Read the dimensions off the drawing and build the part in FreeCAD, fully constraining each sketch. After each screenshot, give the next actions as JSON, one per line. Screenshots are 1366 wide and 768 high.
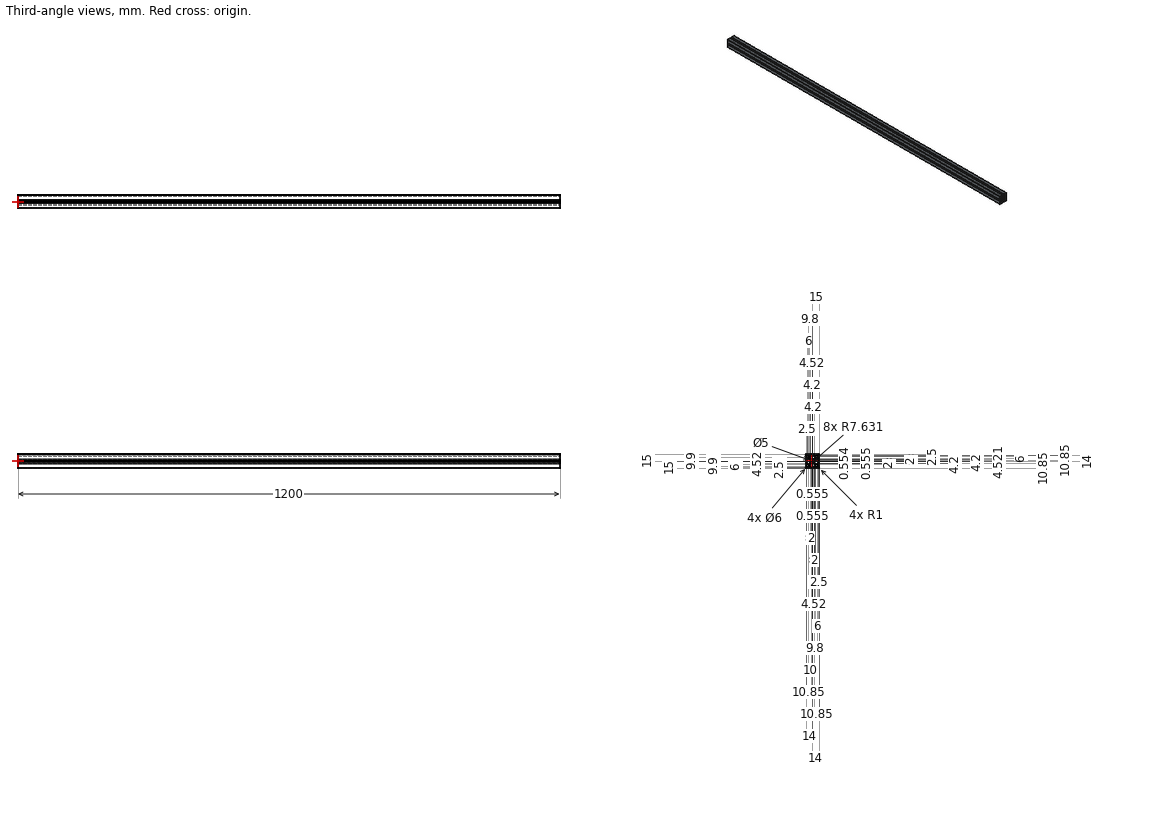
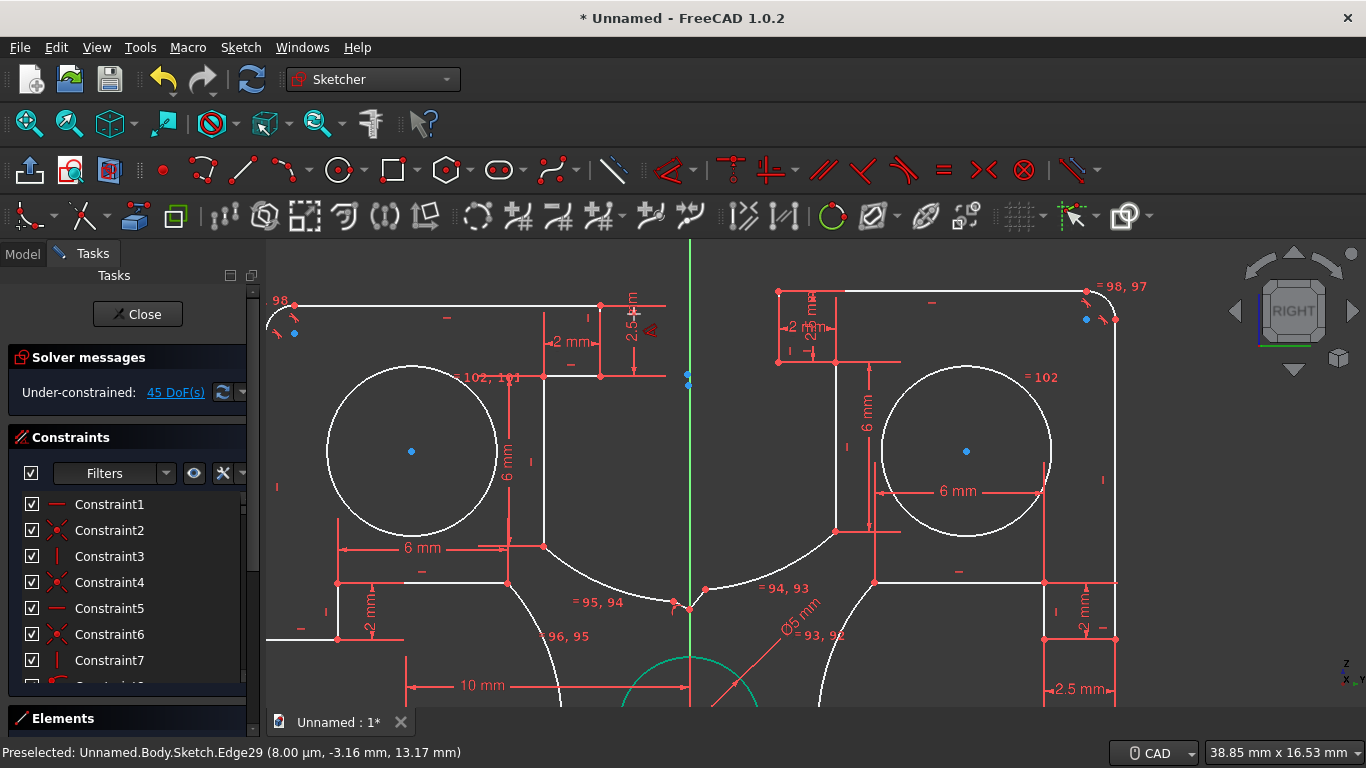
{"action": "left_click", "coordinate": [316, 640]}
{"action": "left_click", "coordinate": [316, 674]}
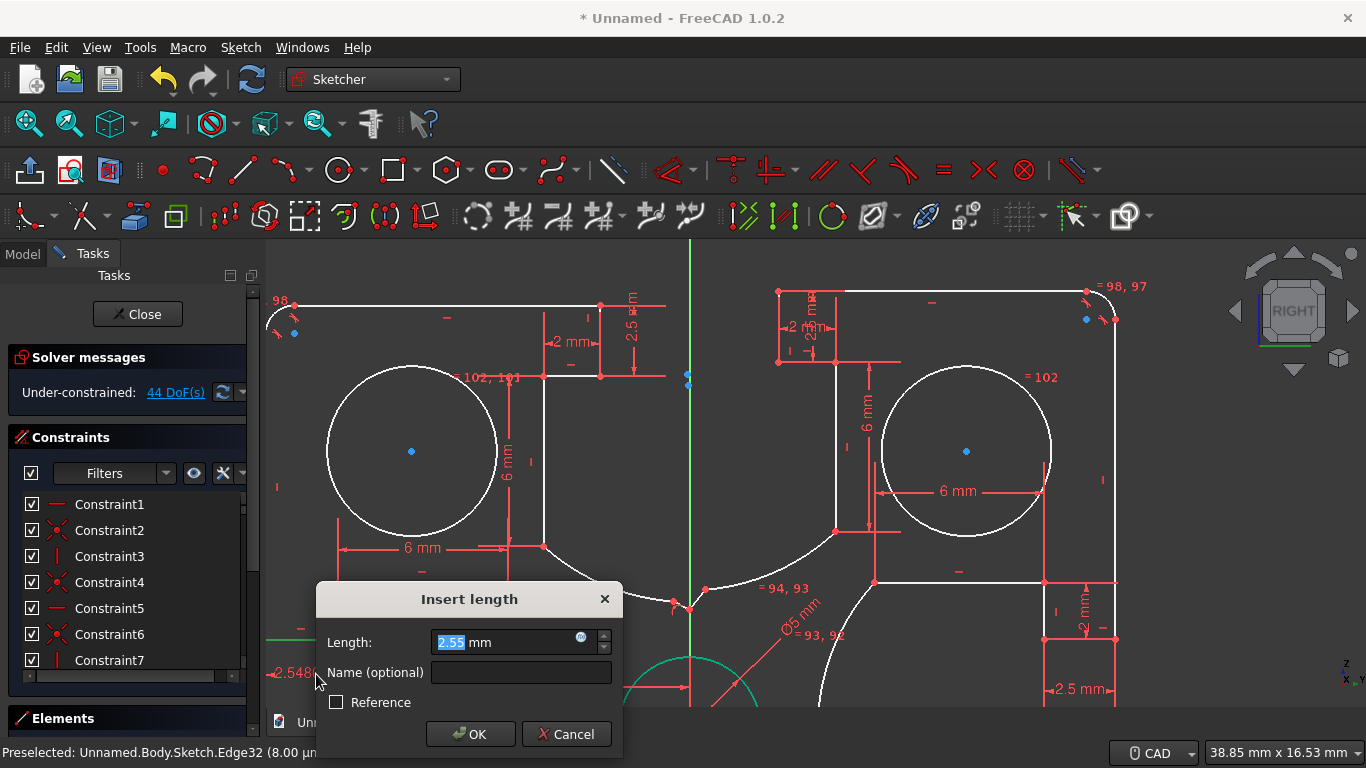
{"action": "type", "text": "2.5"}
{"action": "key", "text": "Return"}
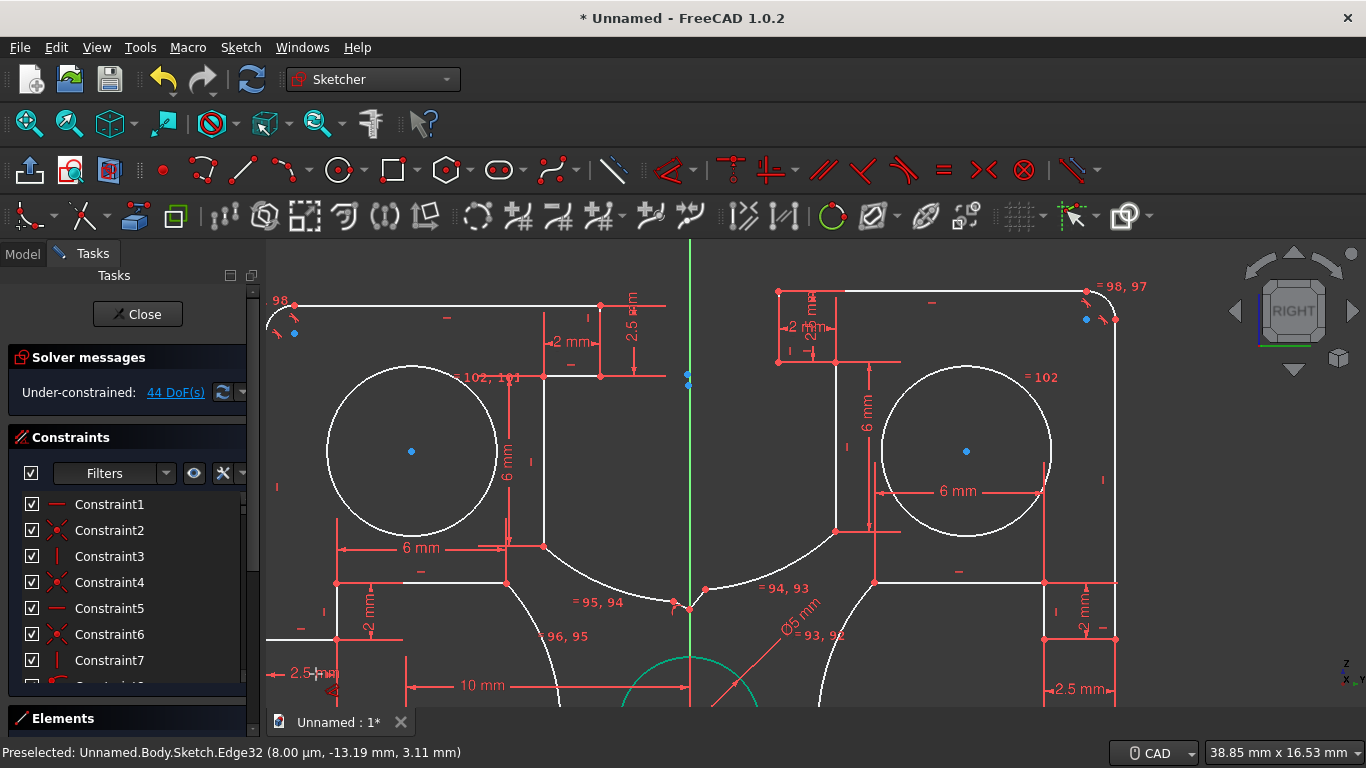
{"action": "scroll", "coordinate": [781, 325], "scroll_direction": "down", "scroll_amount": 5}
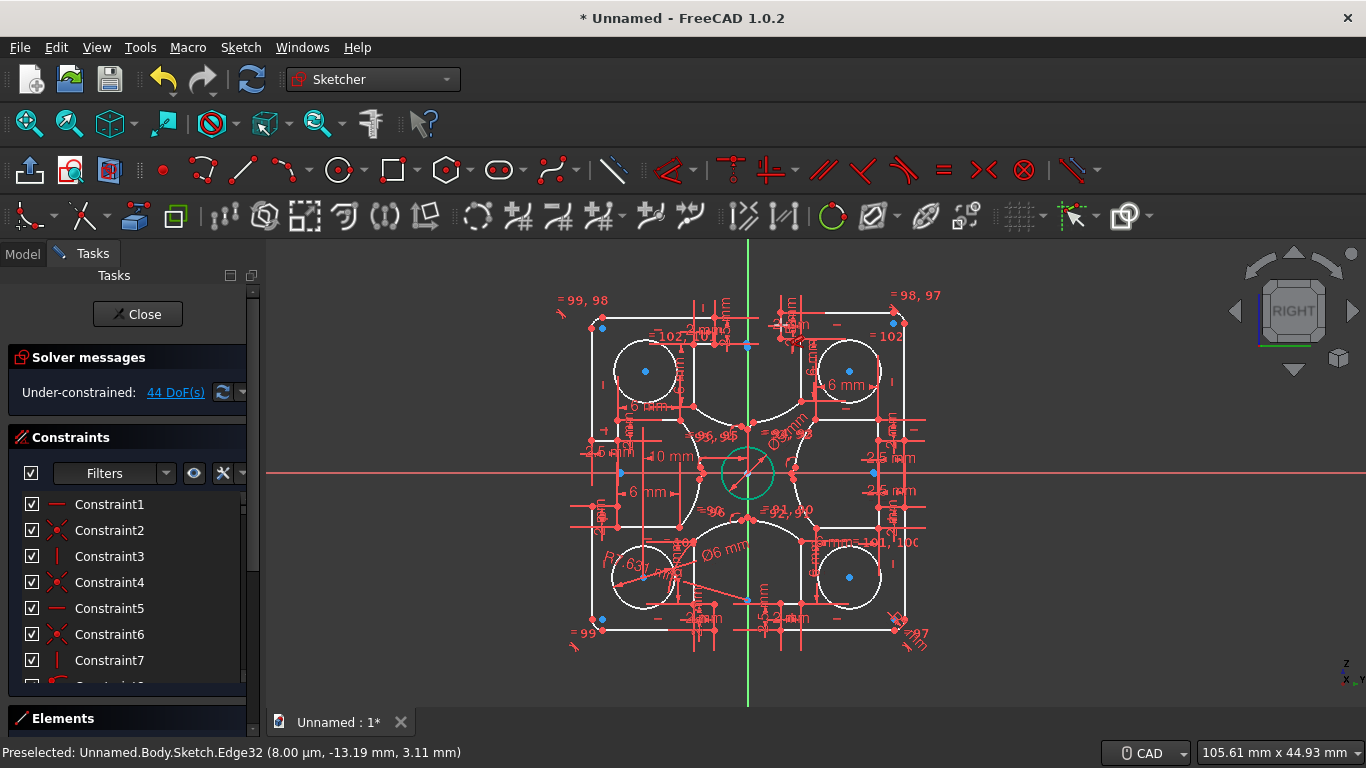
{"action": "scroll", "coordinate": [610, 506], "scroll_direction": "up", "scroll_amount": 4}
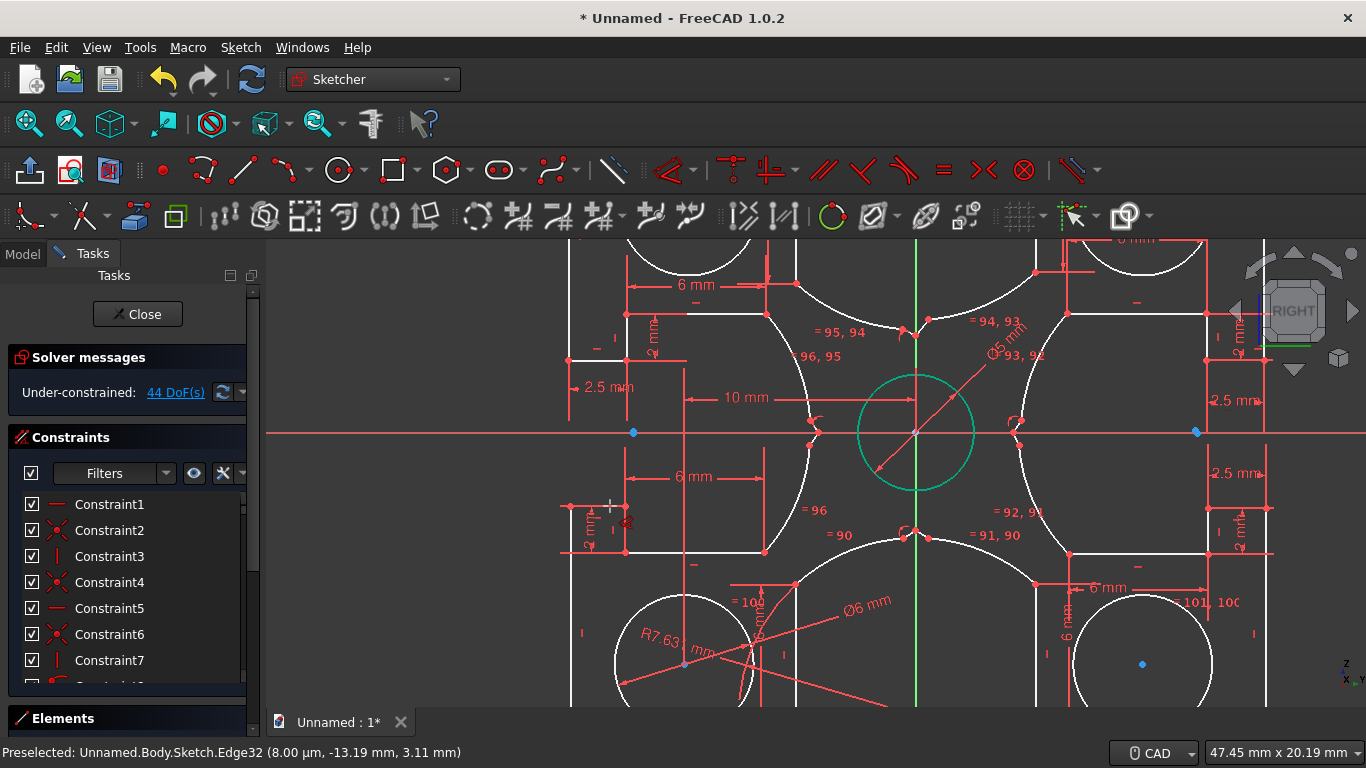
{"action": "left_click", "coordinate": [609, 506]}
{"action": "left_click", "coordinate": [598, 472]}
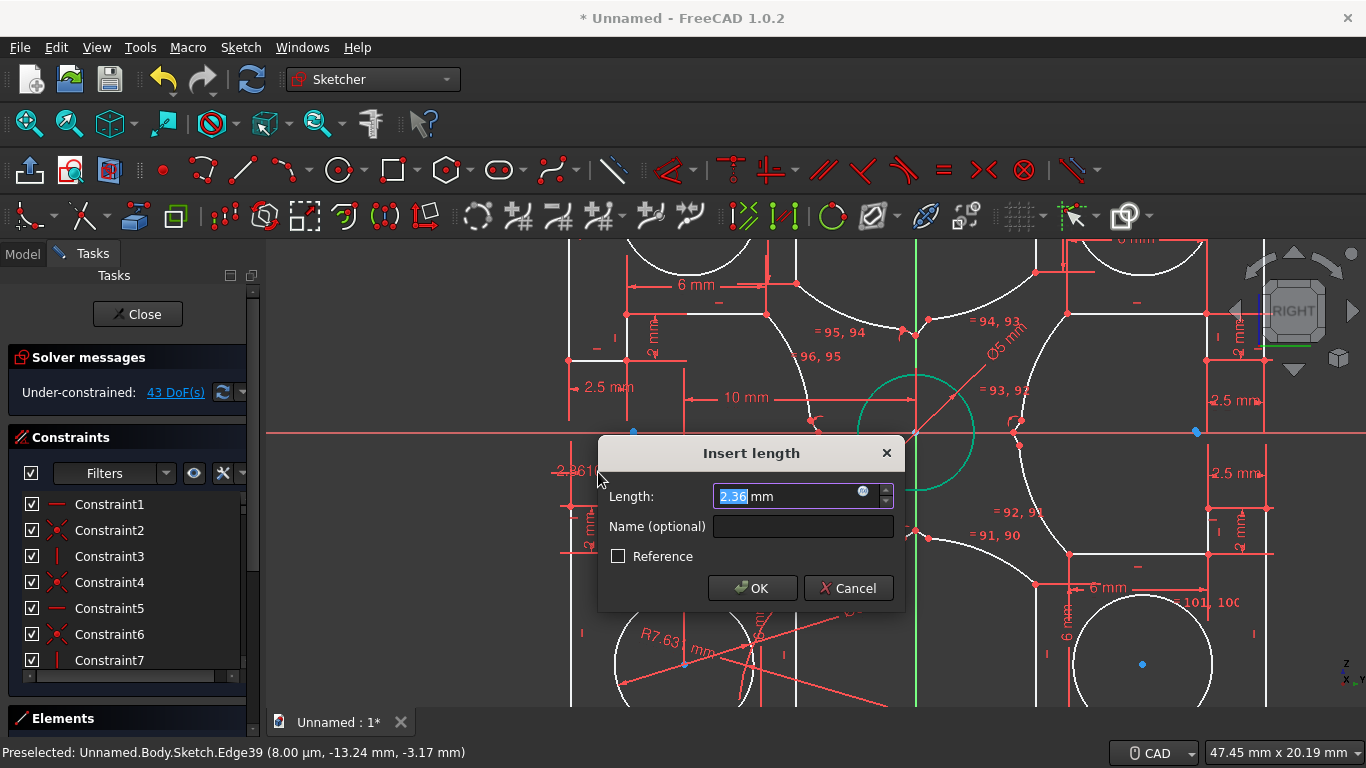
{"action": "type", "text": "2.5"}
{"action": "key", "text": "Return"}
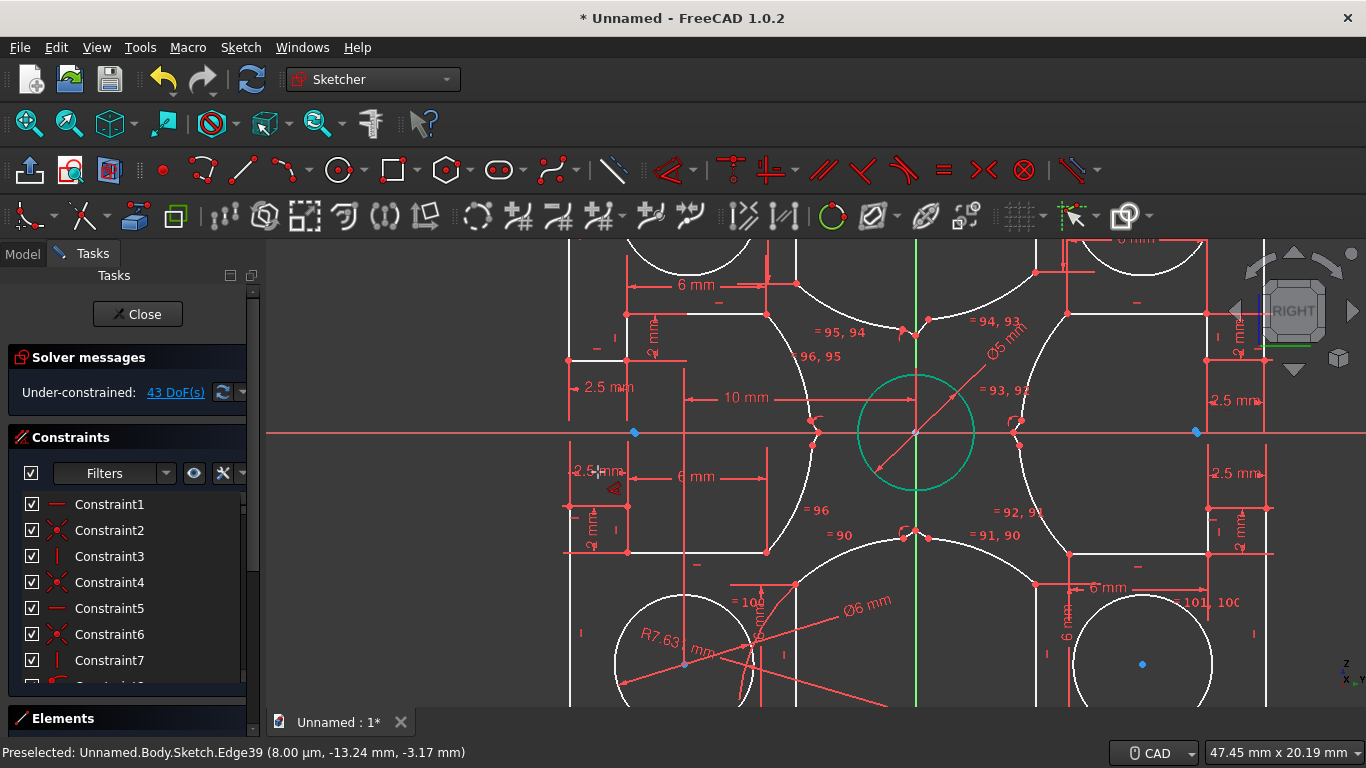
{"action": "scroll", "coordinate": [610, 506], "scroll_direction": "down", "scroll_amount": 4}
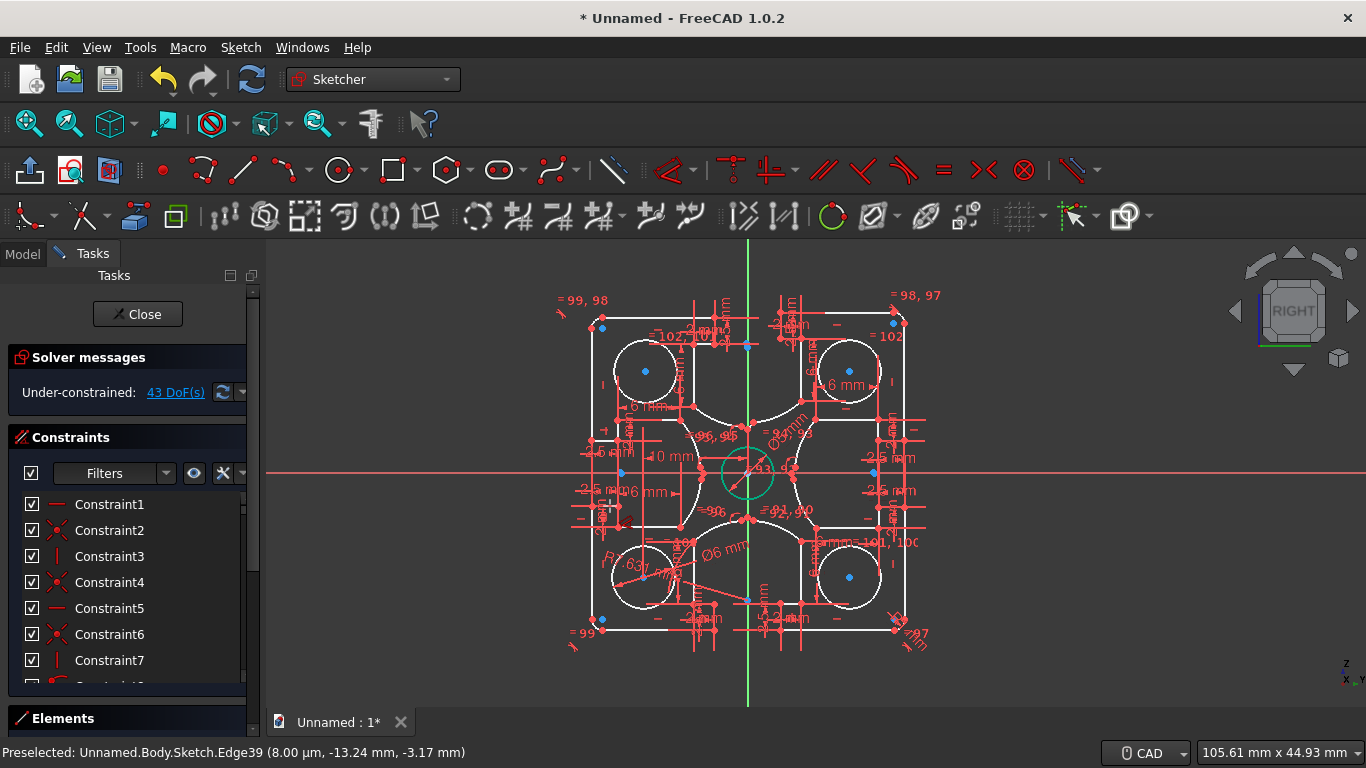
{"action": "left_click", "coordinate": [603, 630]}
{"action": "left_click", "coordinate": [675, 664]}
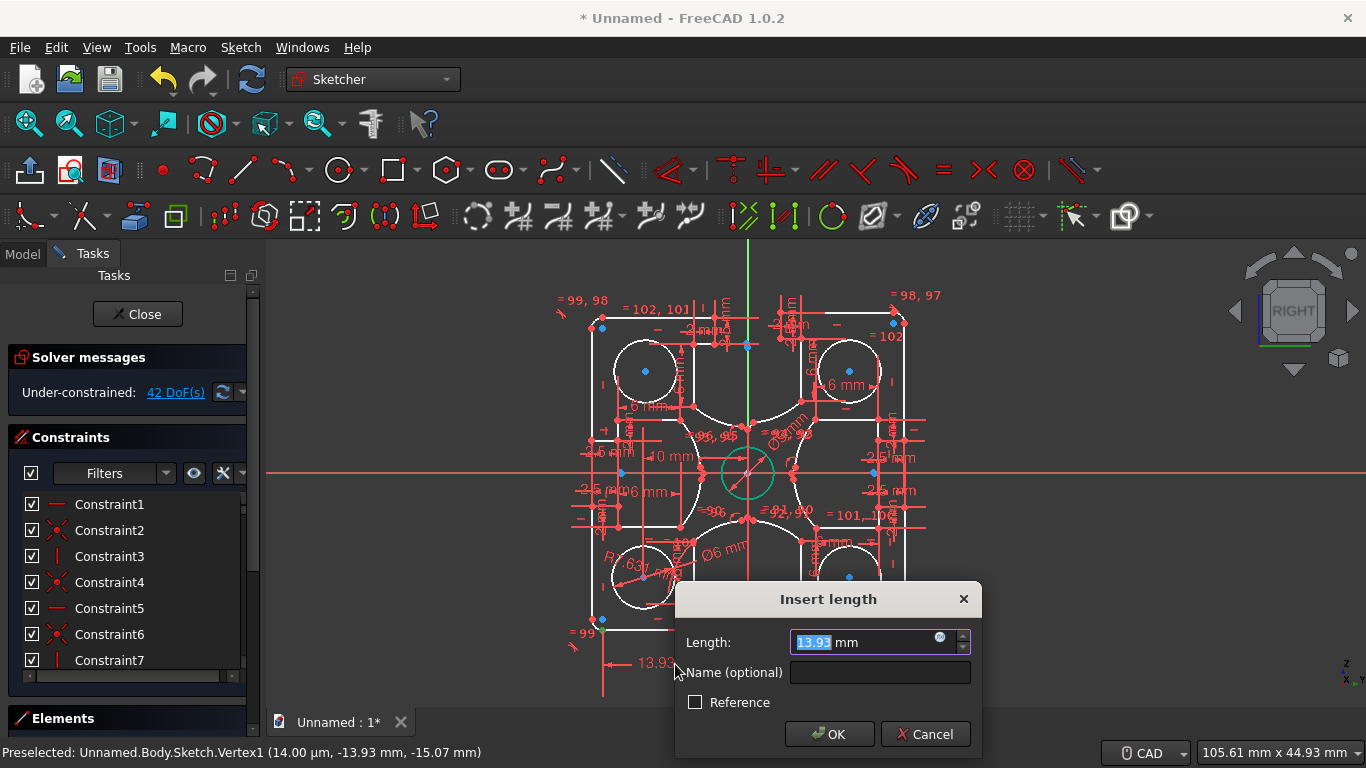
{"action": "type", "text": "14"}
{"action": "key", "text": "Return"}